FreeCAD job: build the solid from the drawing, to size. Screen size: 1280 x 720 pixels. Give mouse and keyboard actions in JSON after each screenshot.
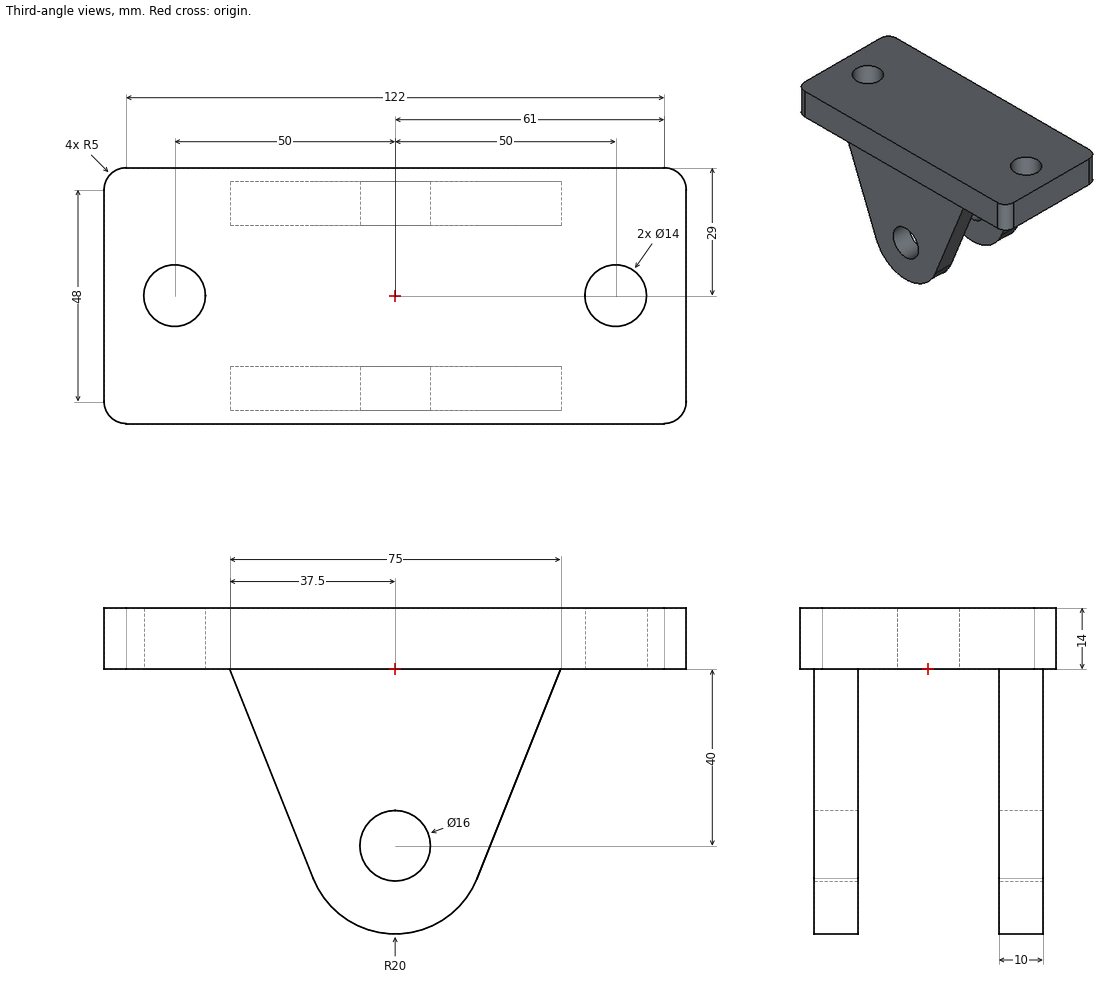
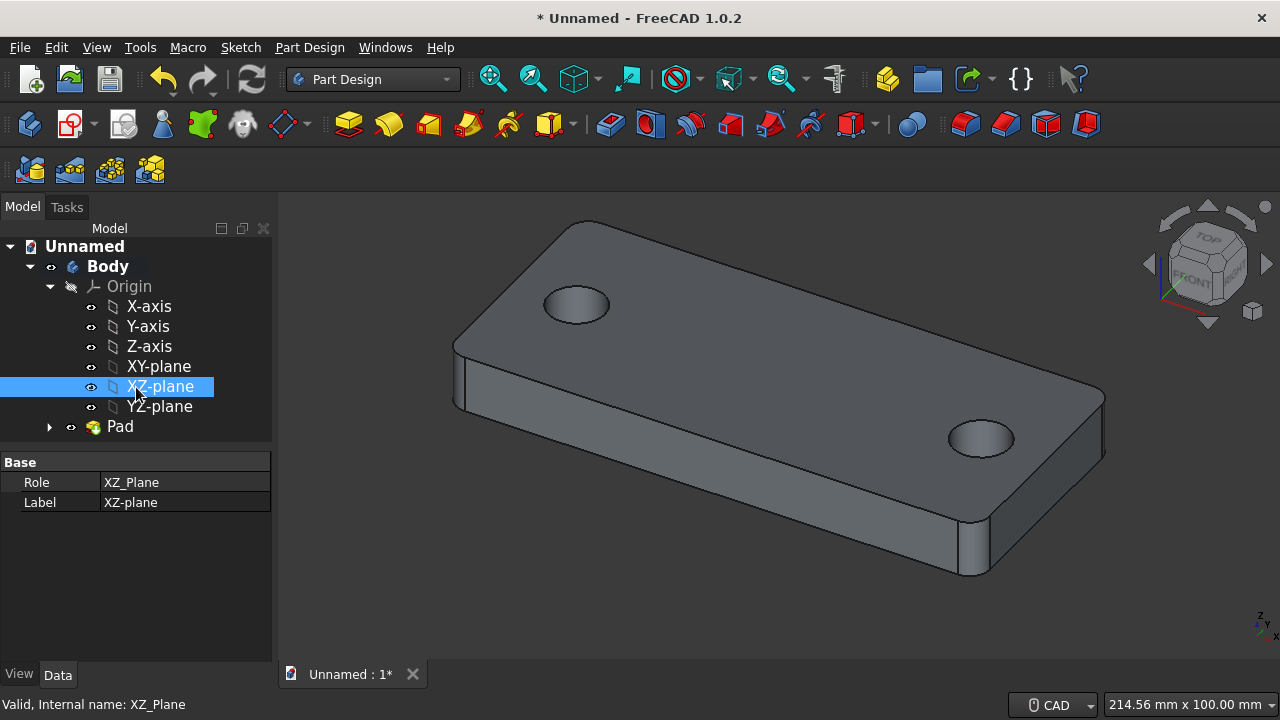
{"action": "left_click", "coordinate": [284, 124]}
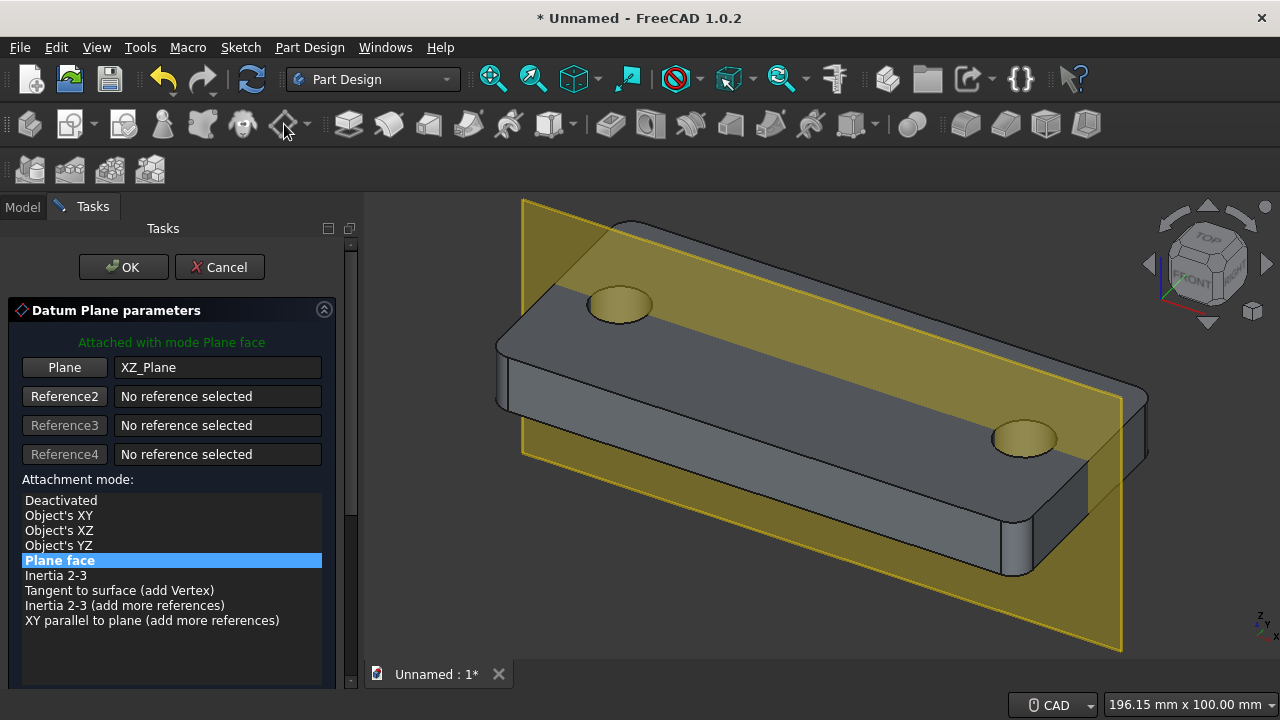
{"action": "scroll", "coordinate": [351, 463], "scroll_direction": "down", "scroll_amount": 3}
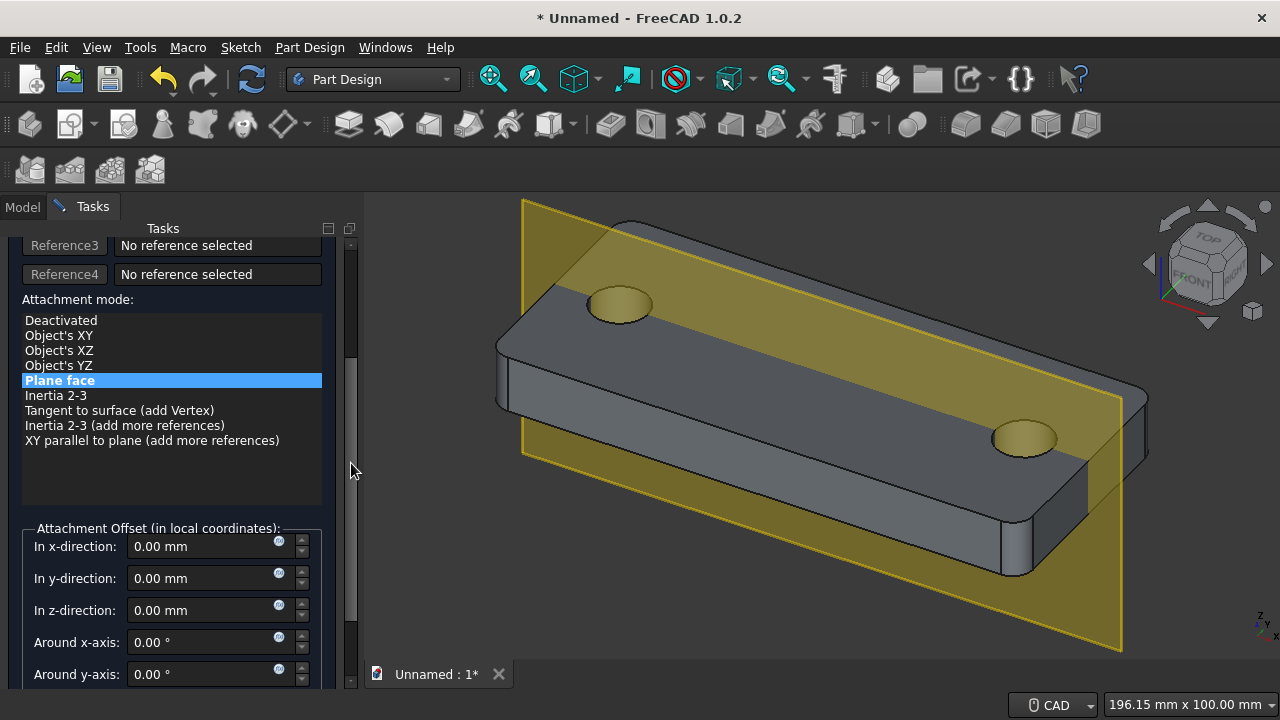
{"action": "triple_click", "coordinate": [210, 610]}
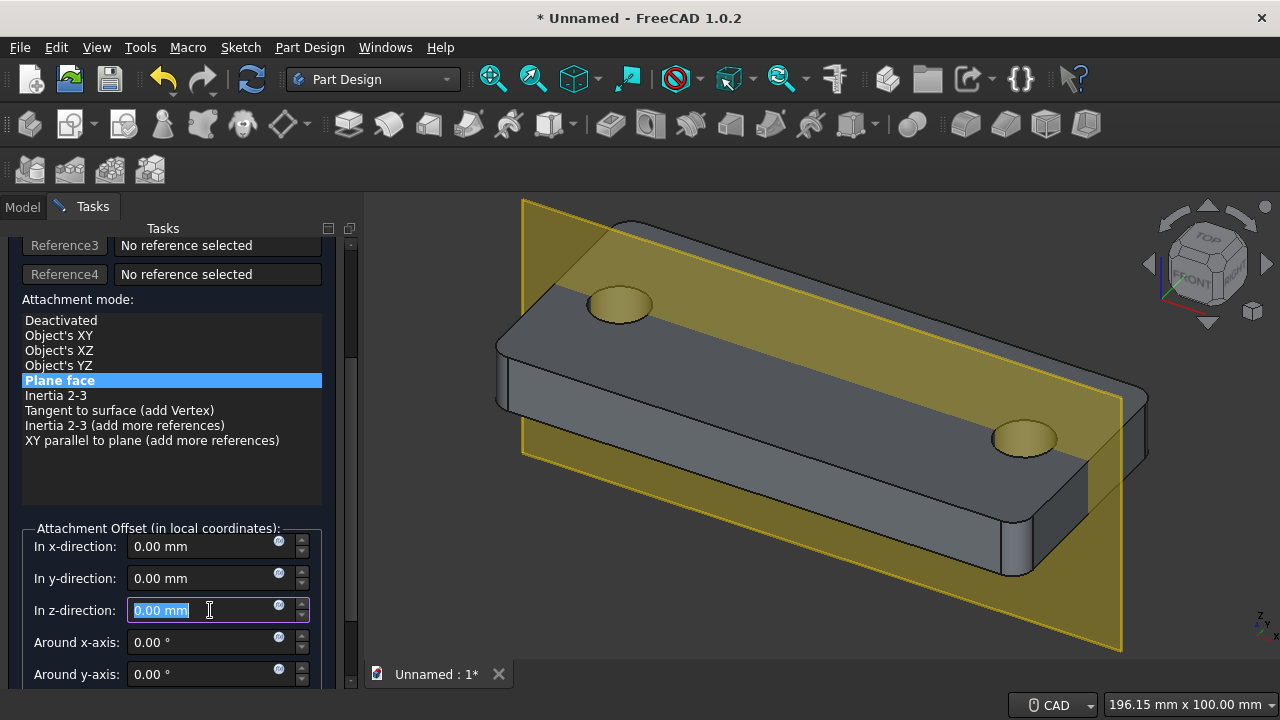
{"action": "type", "text": "-16"}
{"action": "key", "text": "Tab"}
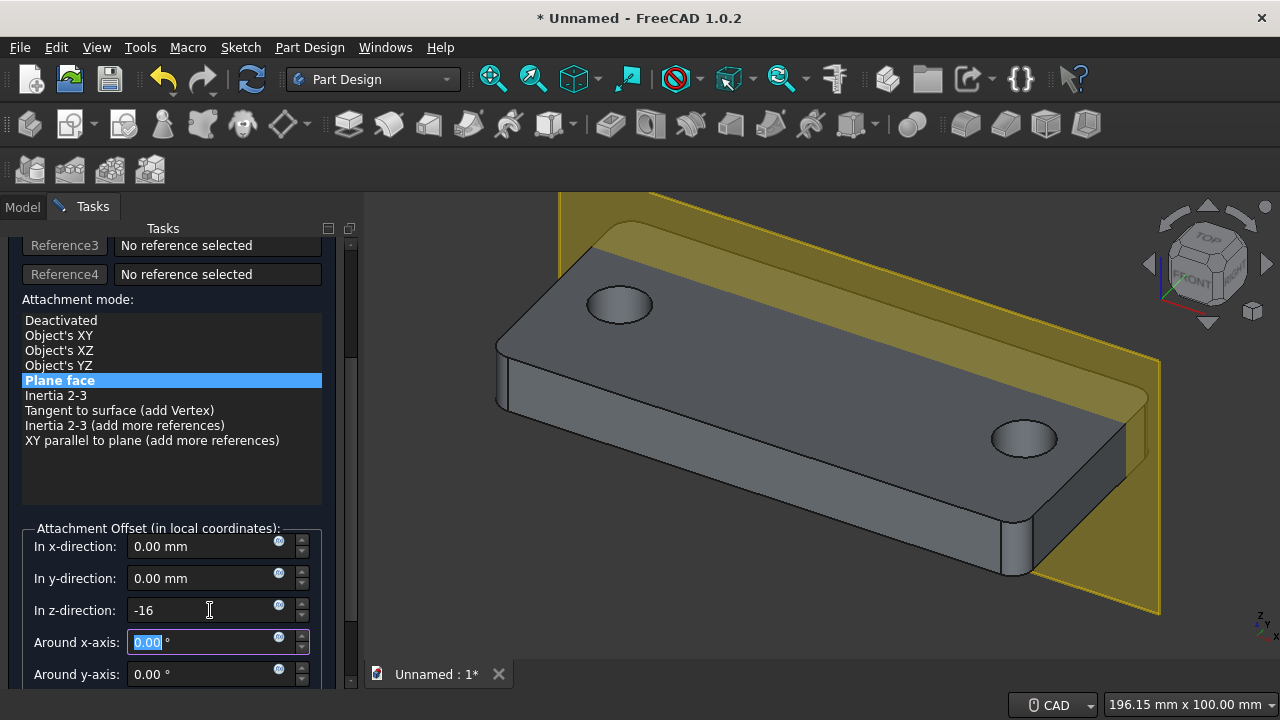
{"action": "scroll", "coordinate": [351, 463], "scroll_direction": "up", "scroll_amount": 4}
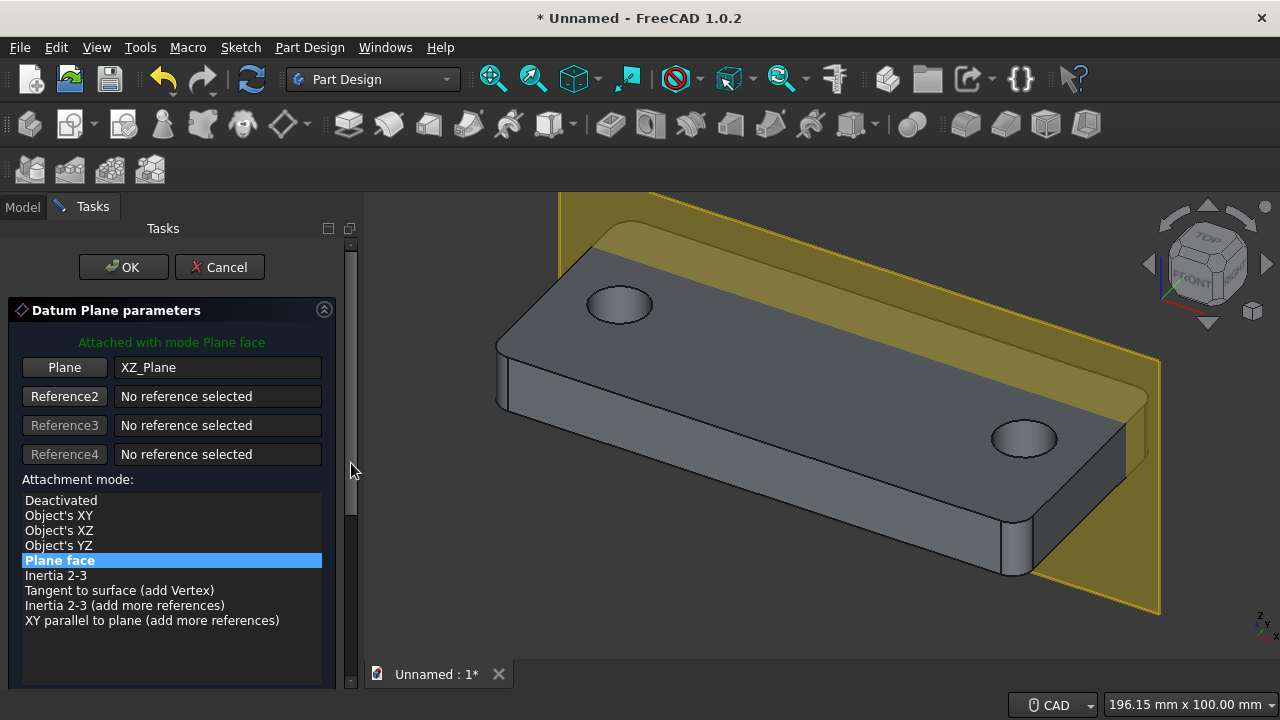
{"action": "left_click", "coordinate": [124, 267]}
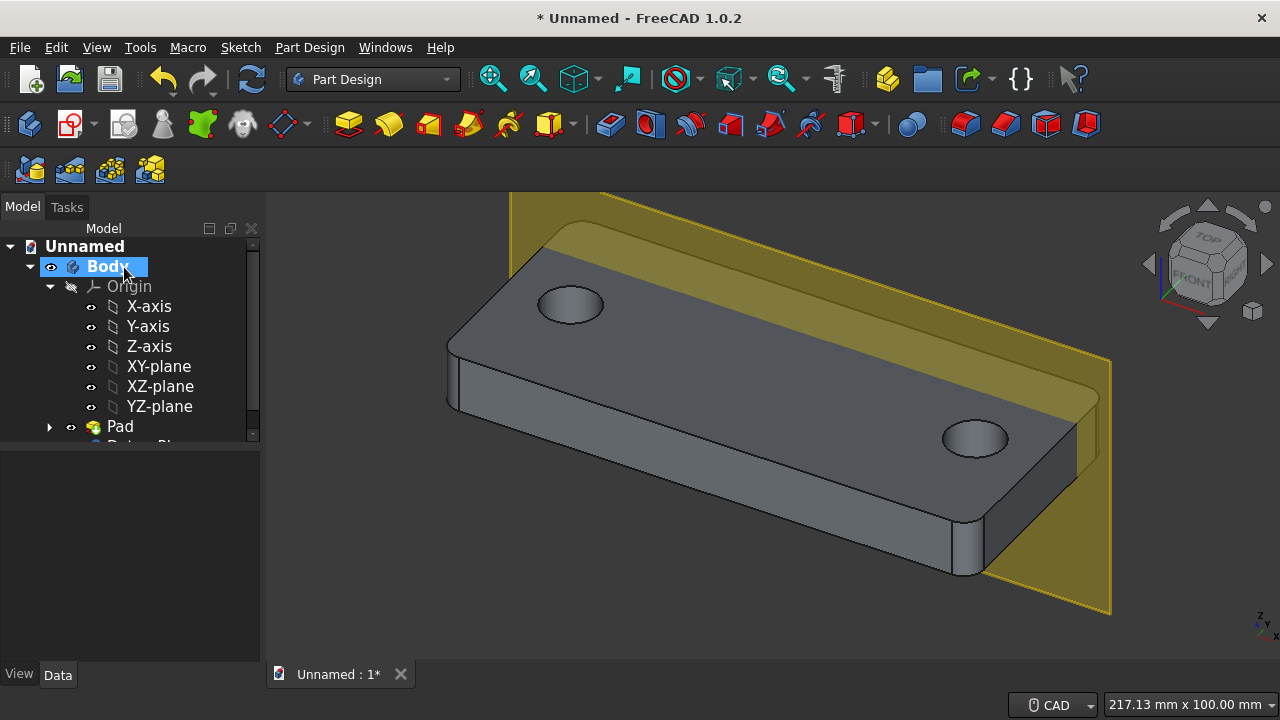
{"action": "scroll", "coordinate": [100, 342], "scroll_direction": "down", "scroll_amount": 3}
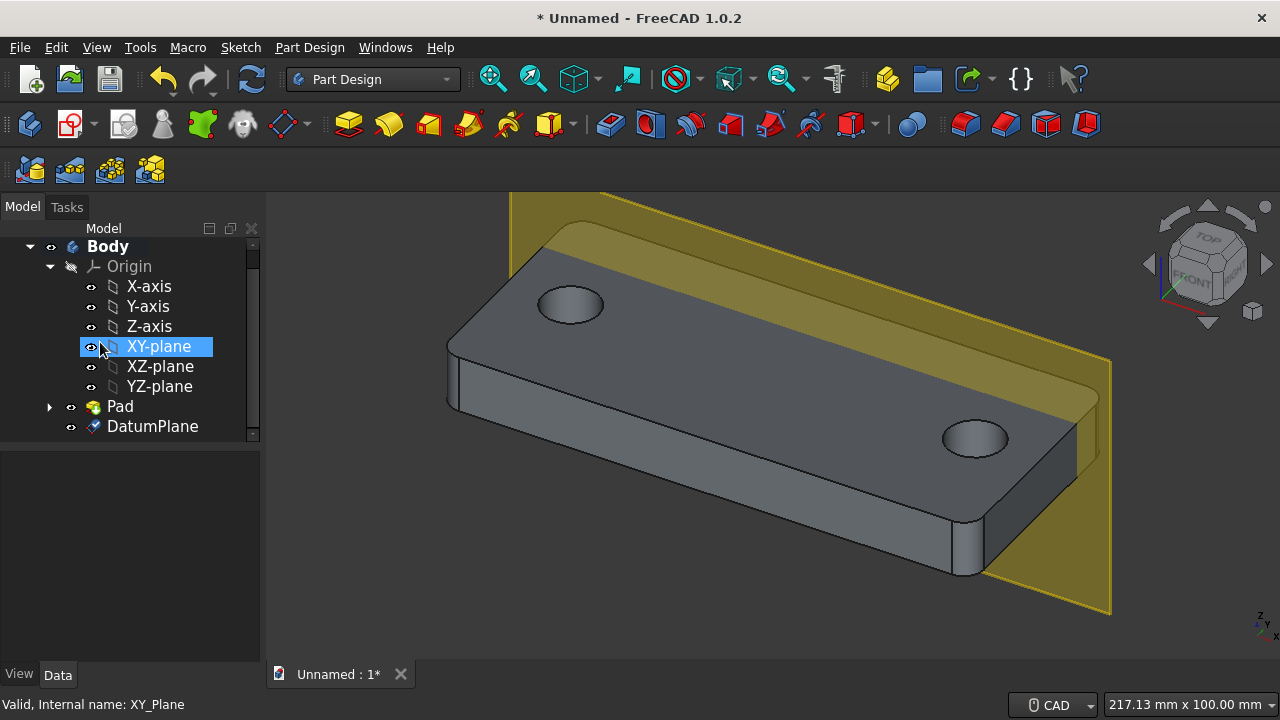
{"action": "left_click", "coordinate": [116, 427]}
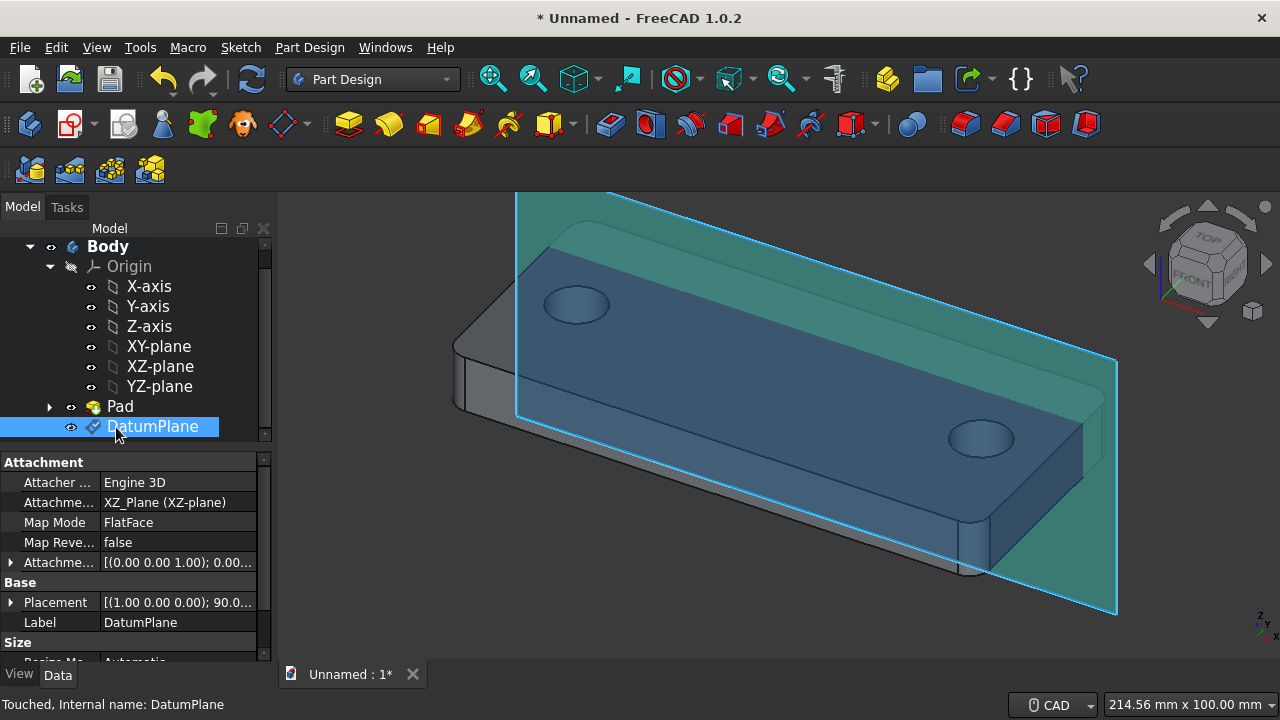
{"action": "left_click", "coordinate": [70, 124]}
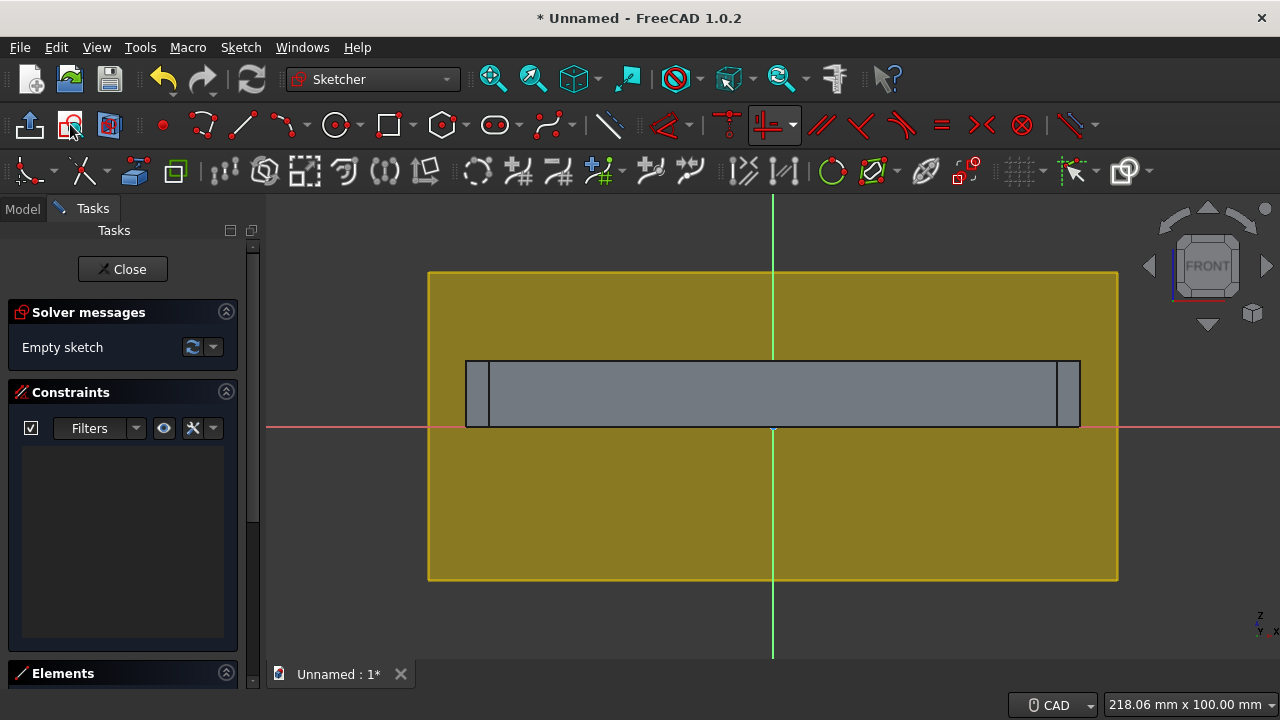
{"action": "left_click", "coordinate": [110, 126]}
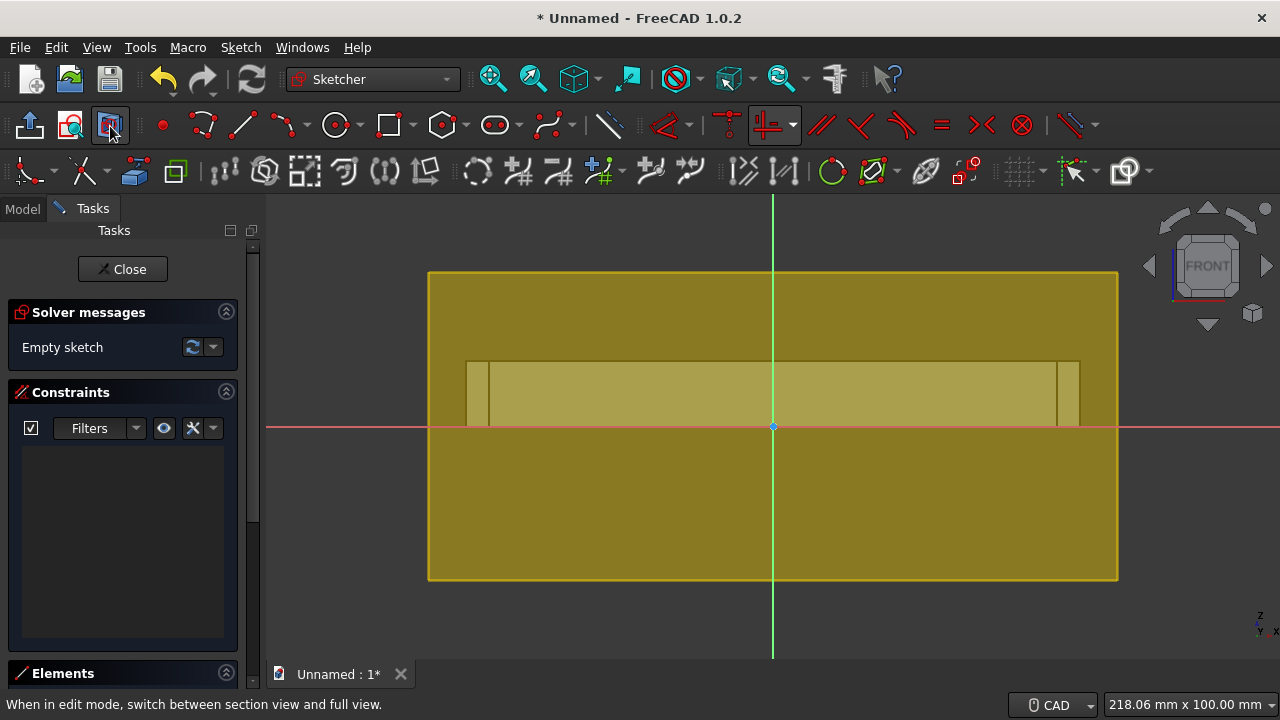
{"action": "scroll", "coordinate": [565, 222], "scroll_direction": "down", "scroll_amount": 2}